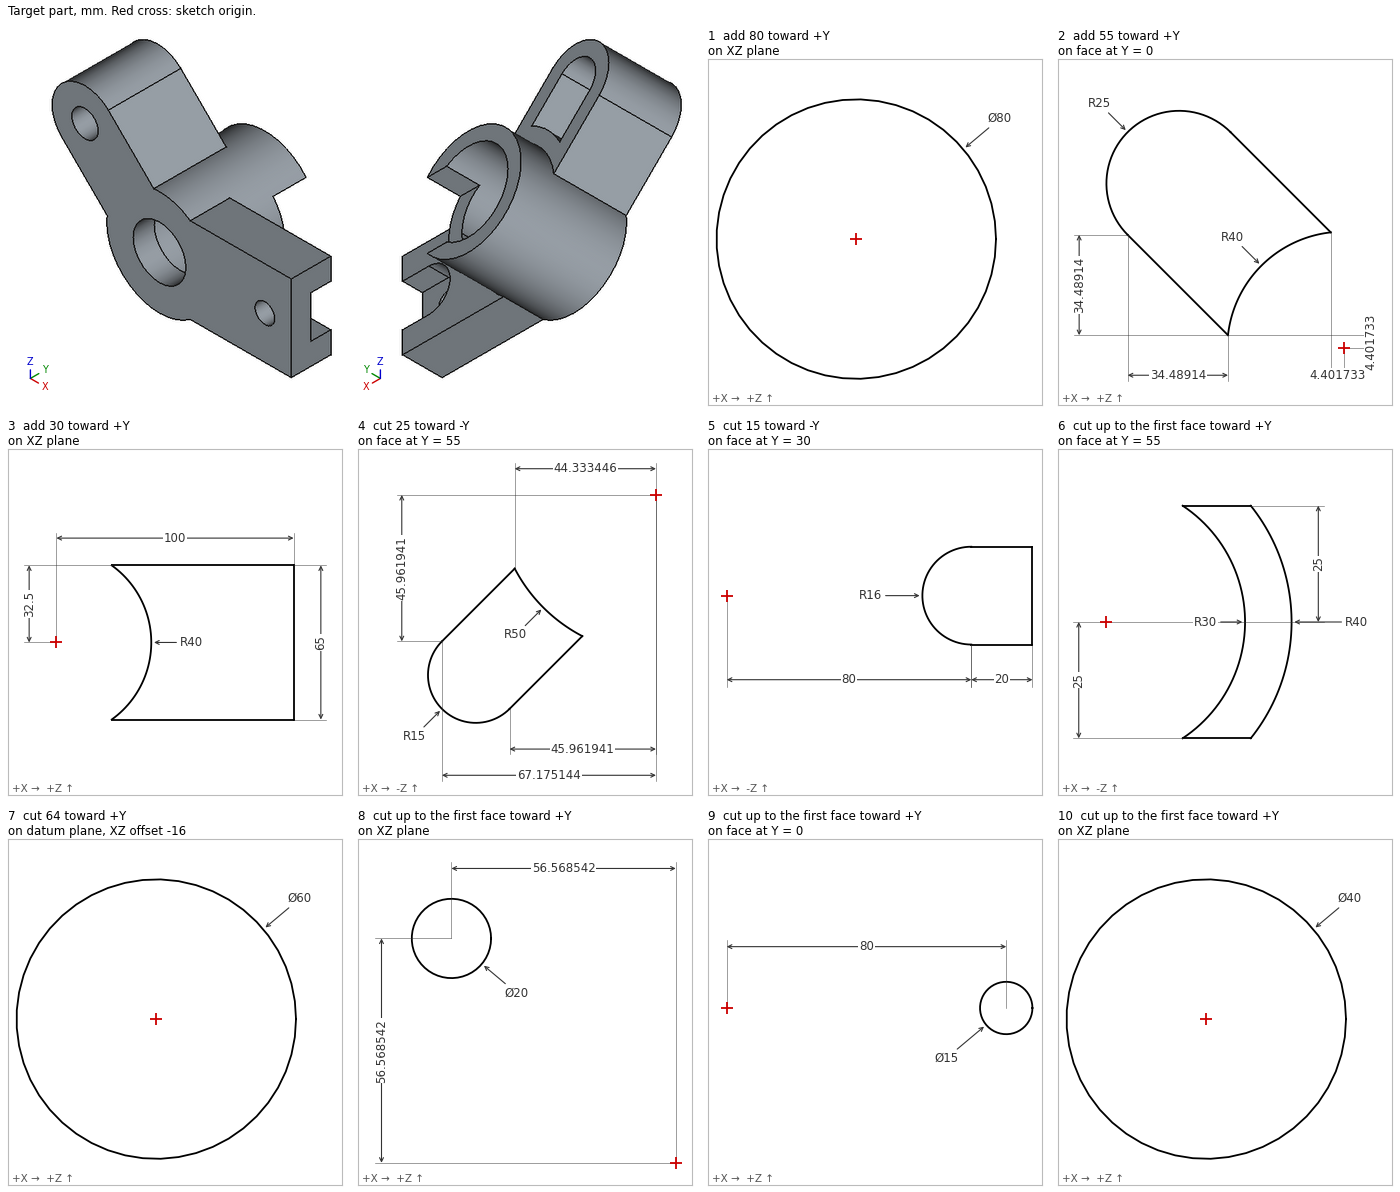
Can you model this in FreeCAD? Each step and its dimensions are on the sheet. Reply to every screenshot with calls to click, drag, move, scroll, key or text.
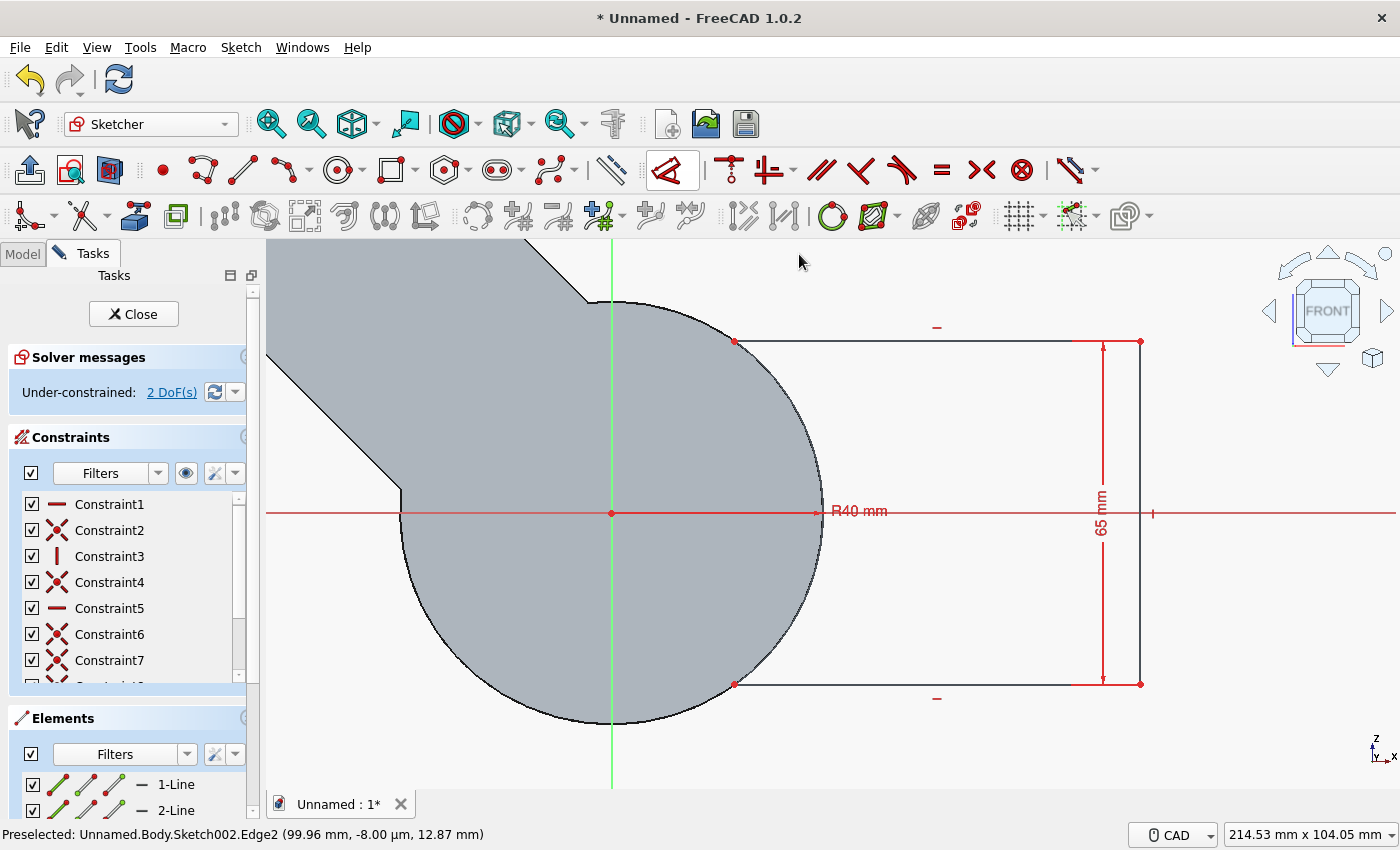
click(1140, 341)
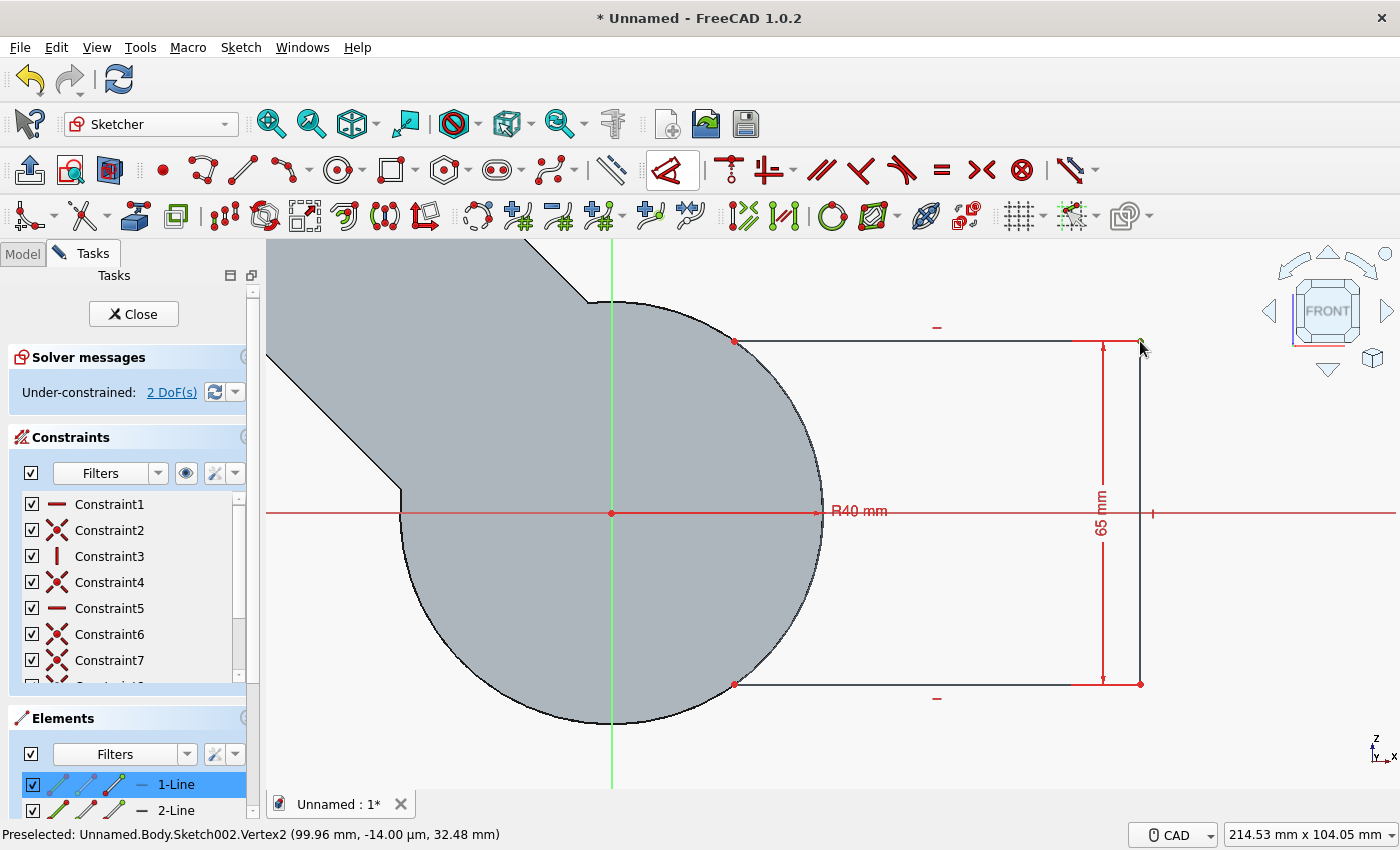
click(694, 170)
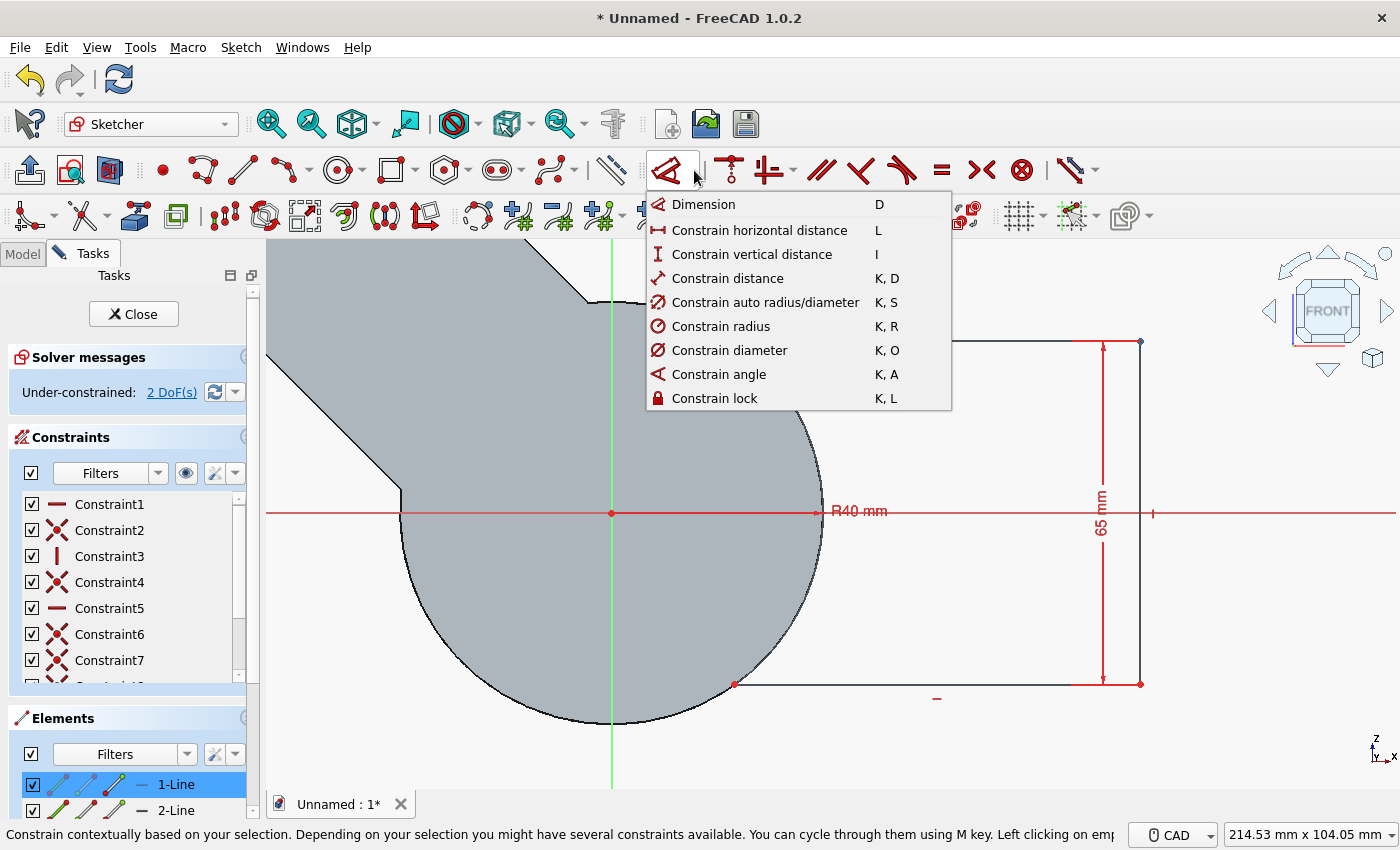
click(799, 230)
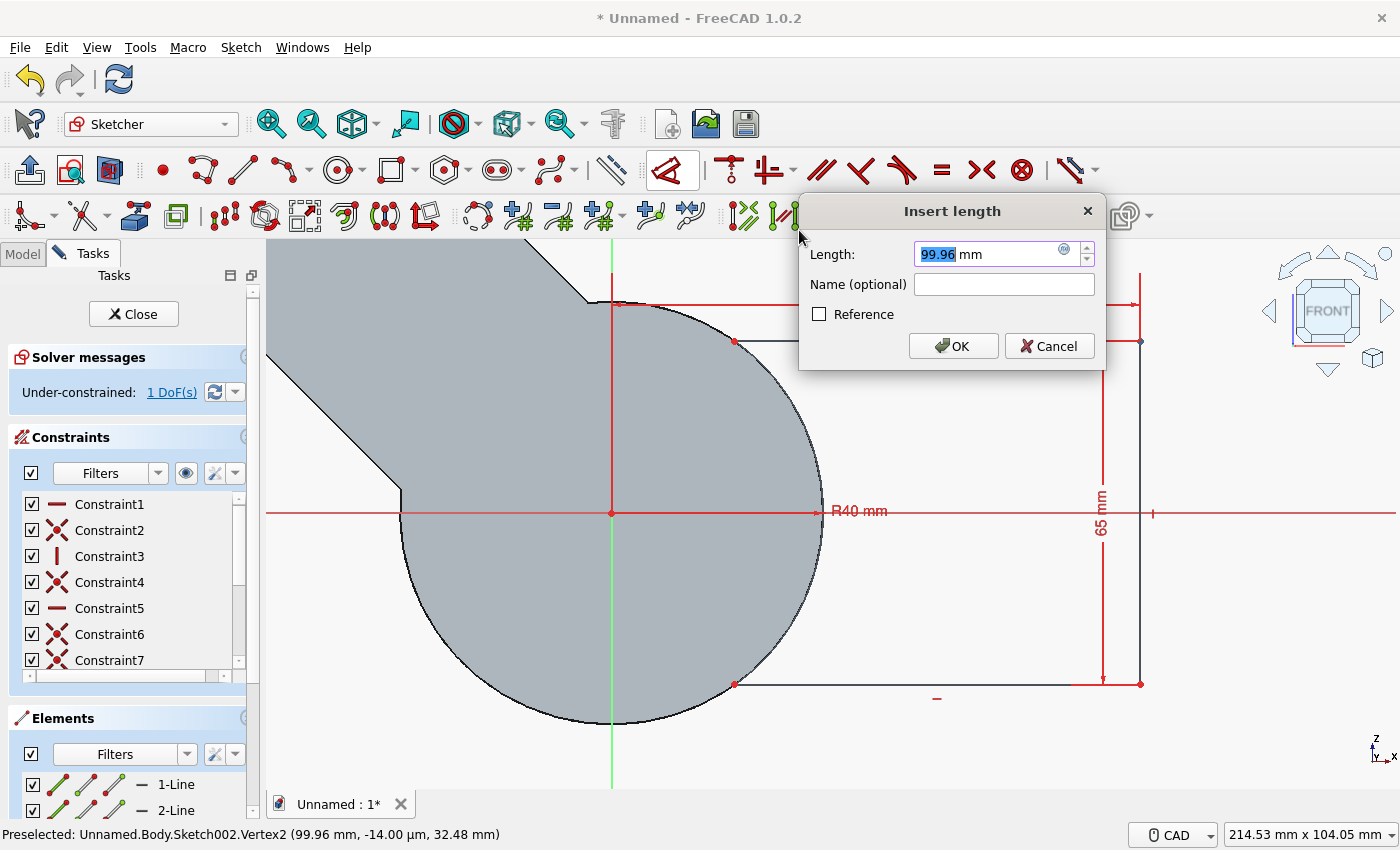
text(100)
key(Return)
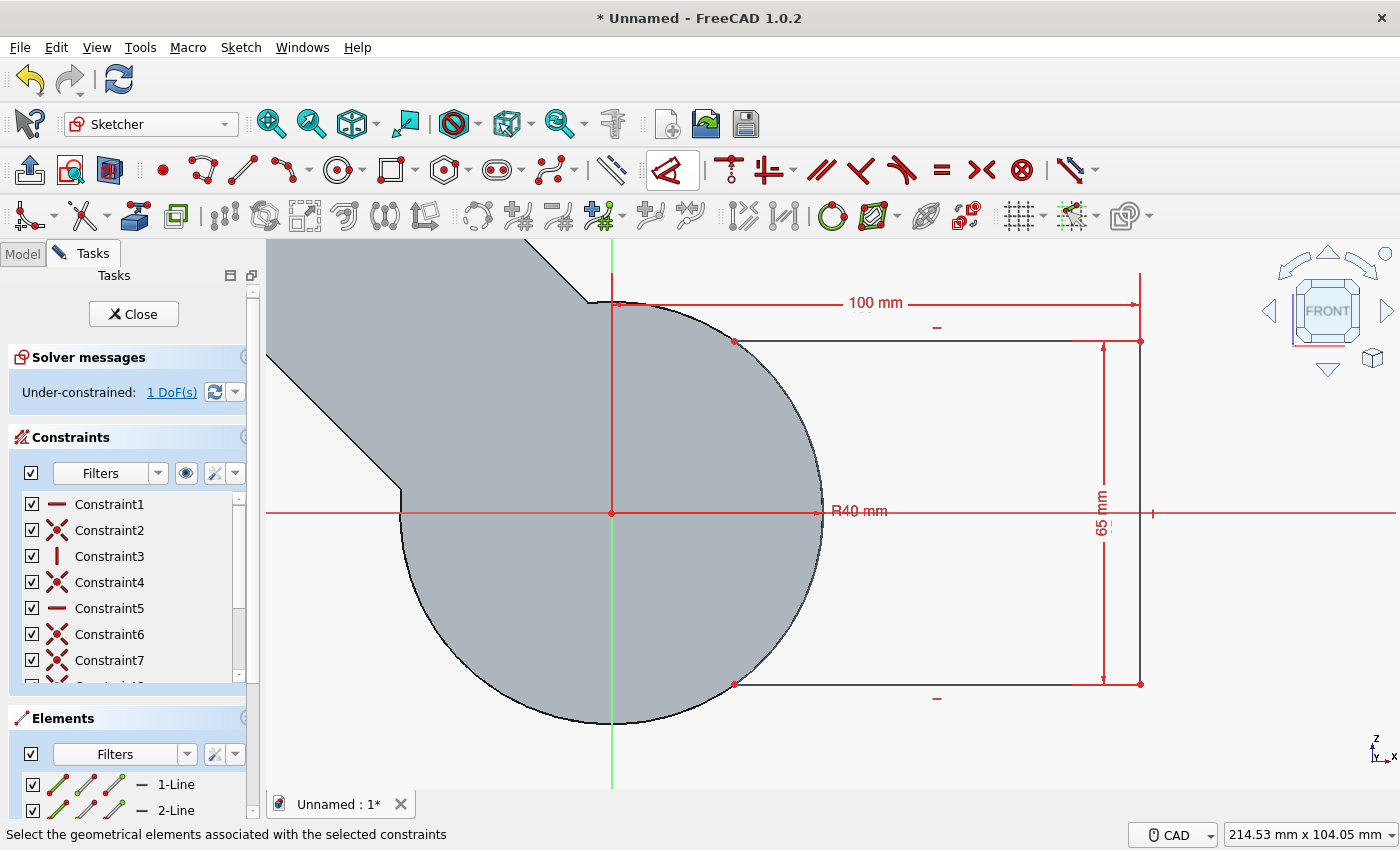
click(735, 341)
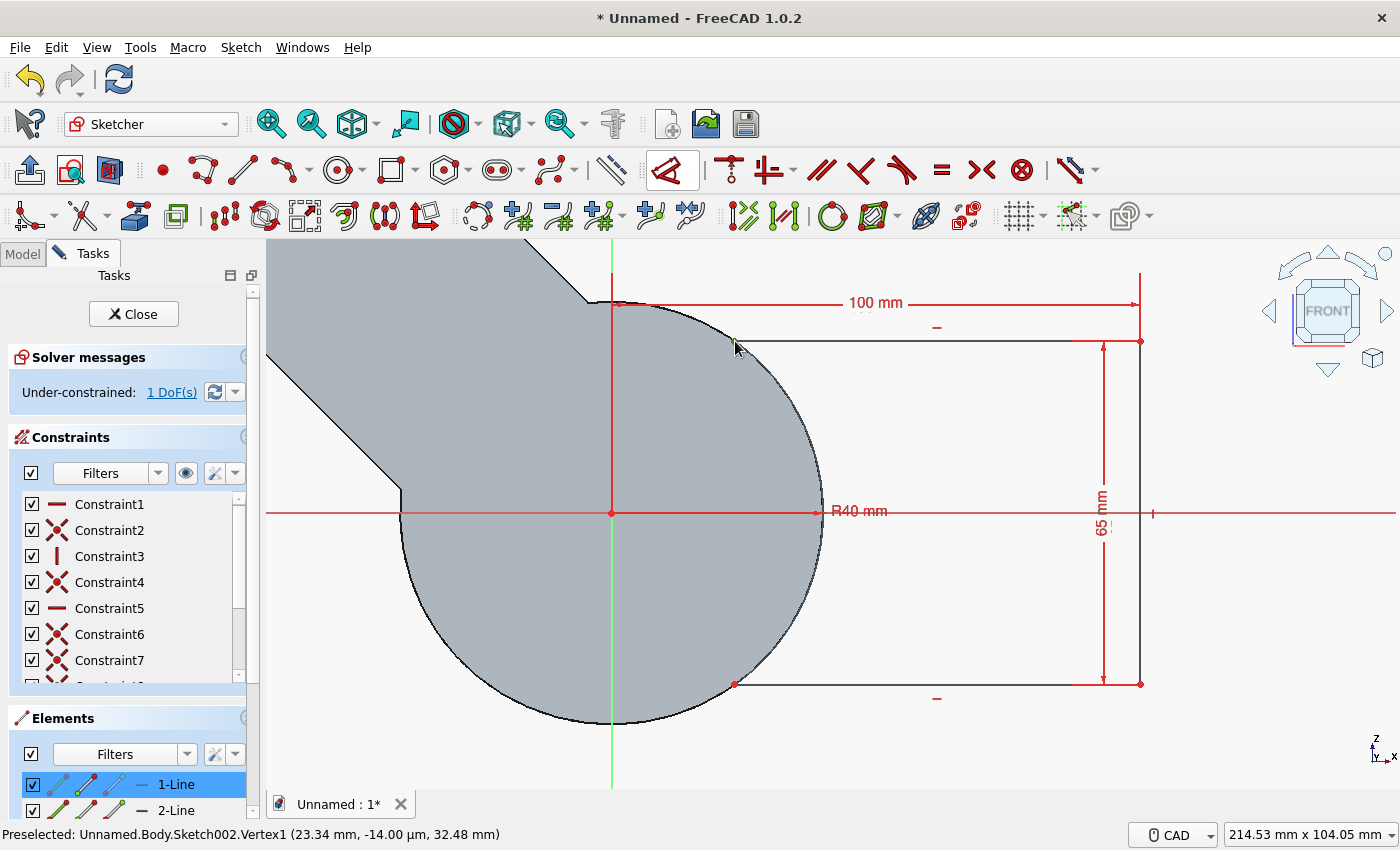
key(i)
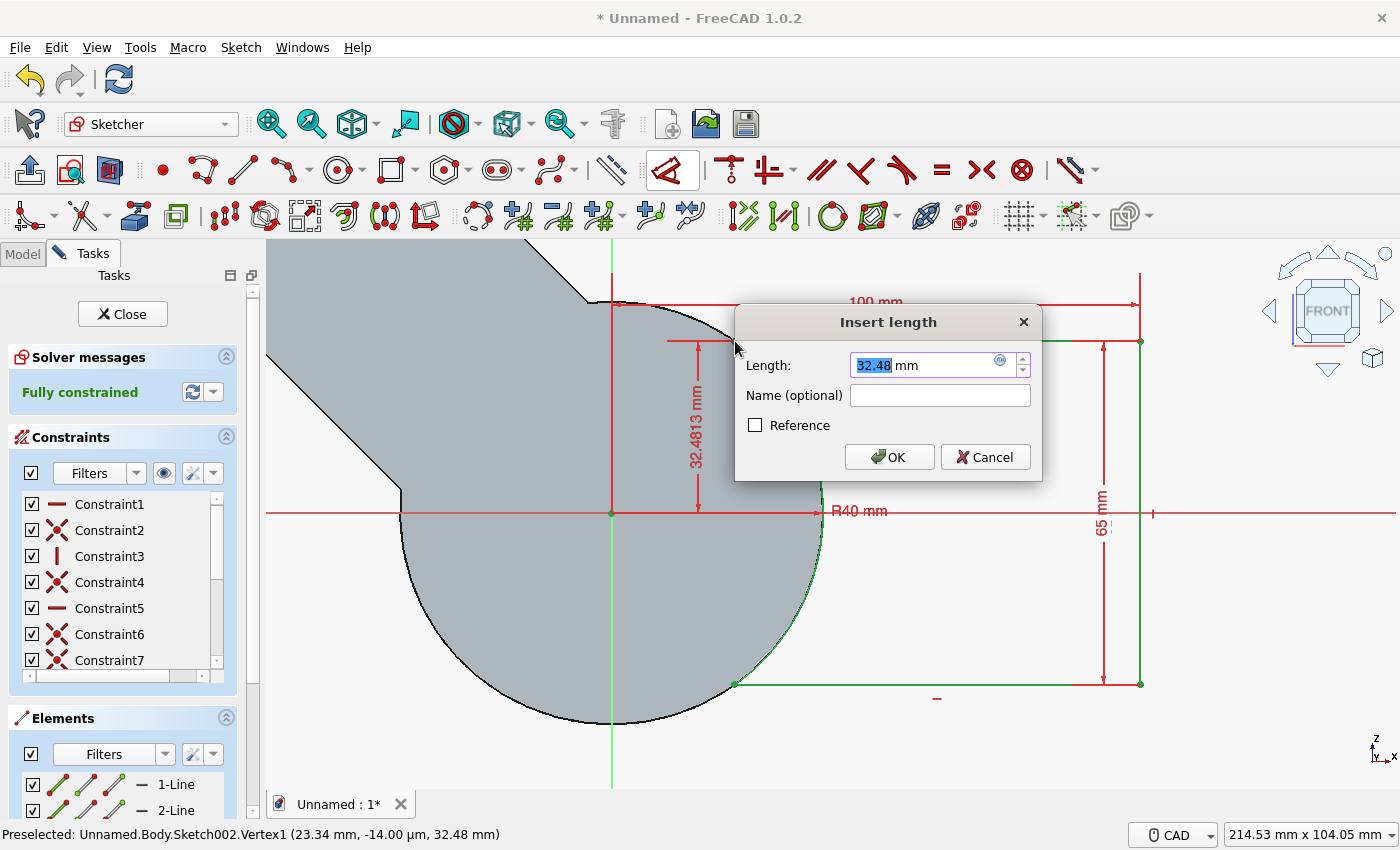
text(32.5)
key(Return)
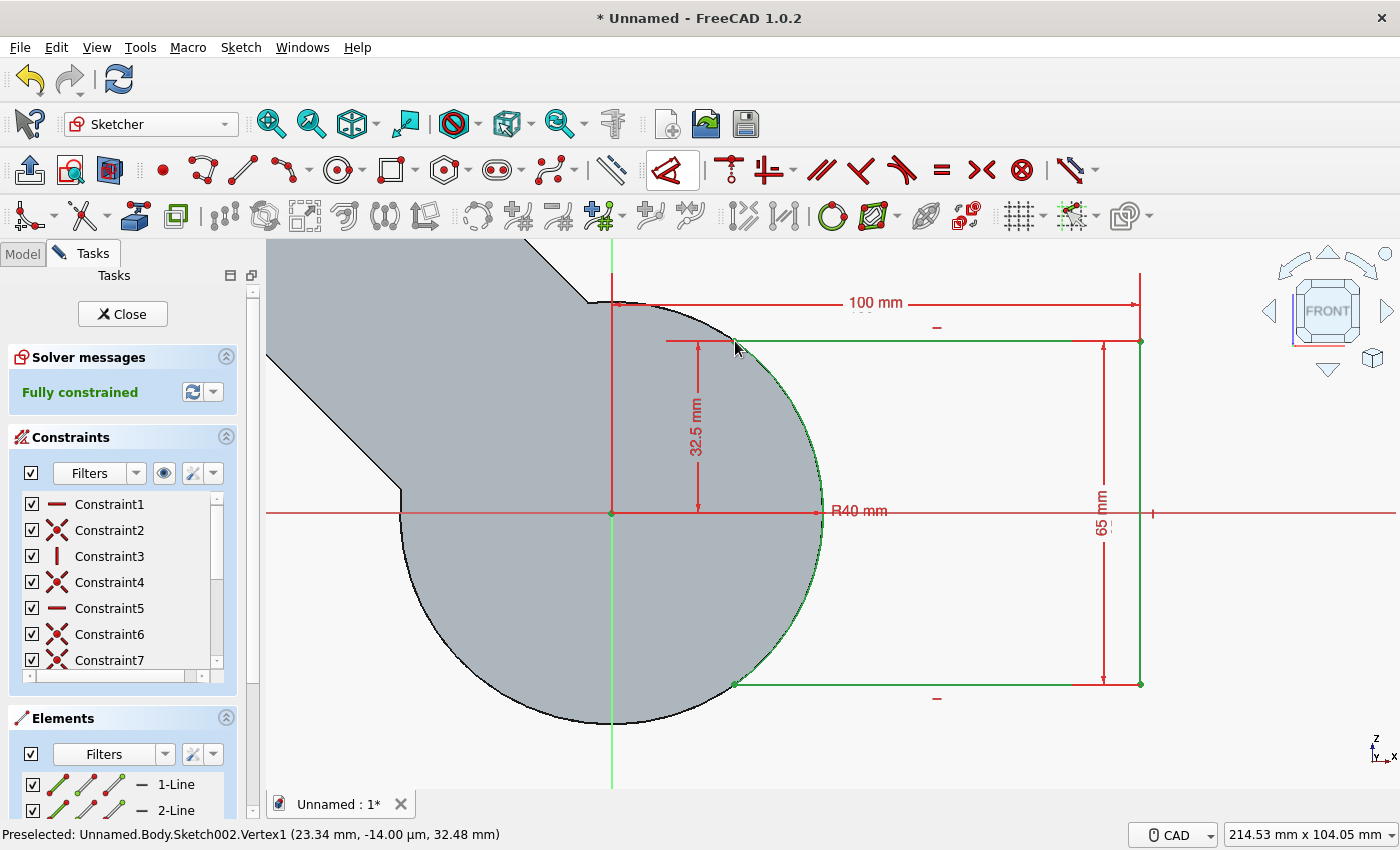
click(123, 314)